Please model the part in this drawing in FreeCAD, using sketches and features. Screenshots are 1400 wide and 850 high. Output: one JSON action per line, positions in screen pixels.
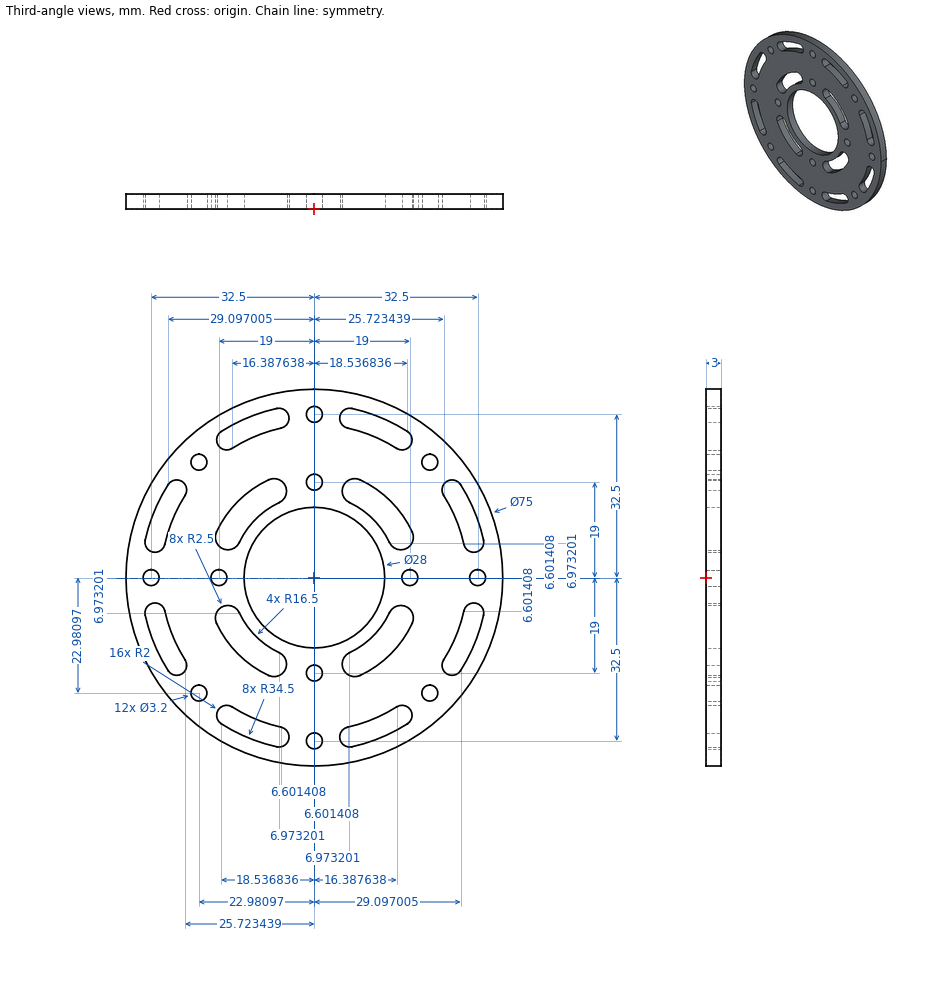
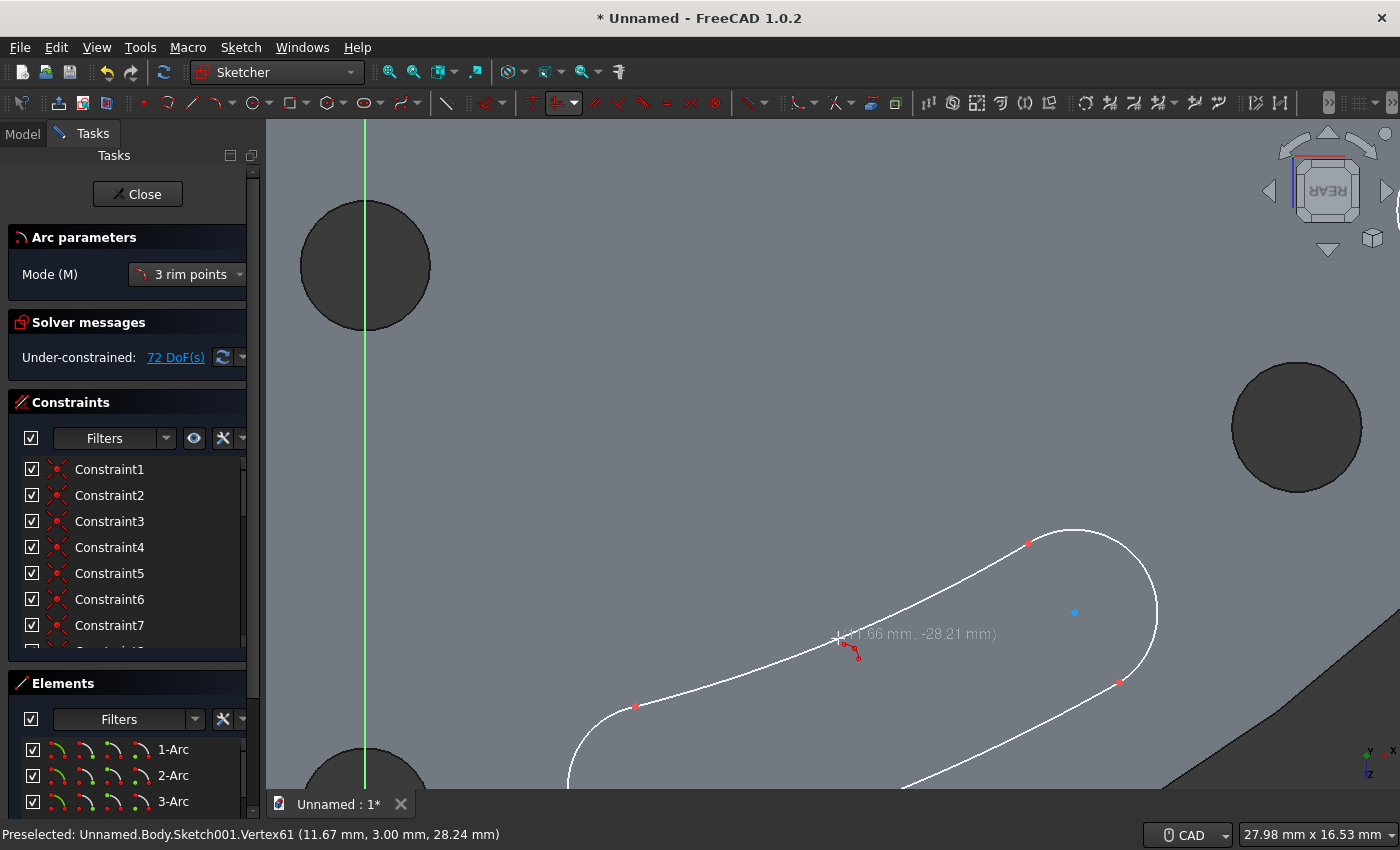
{"action": "scroll", "coordinate": [844, 644], "scroll_direction": "down", "scroll_amount": 9}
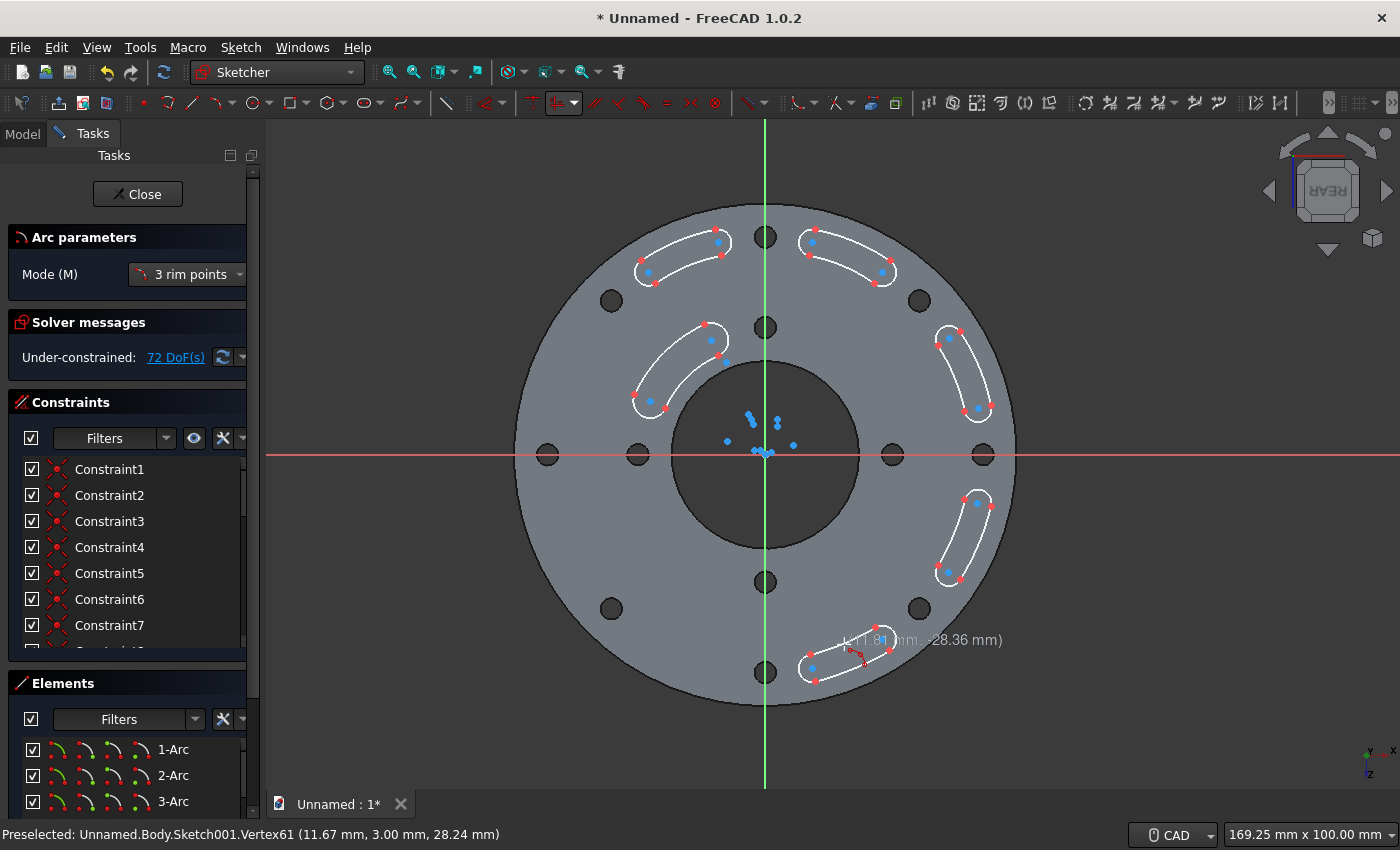
{"action": "left_click", "coordinate": [721, 654]}
{"action": "left_click", "coordinate": [656, 627]}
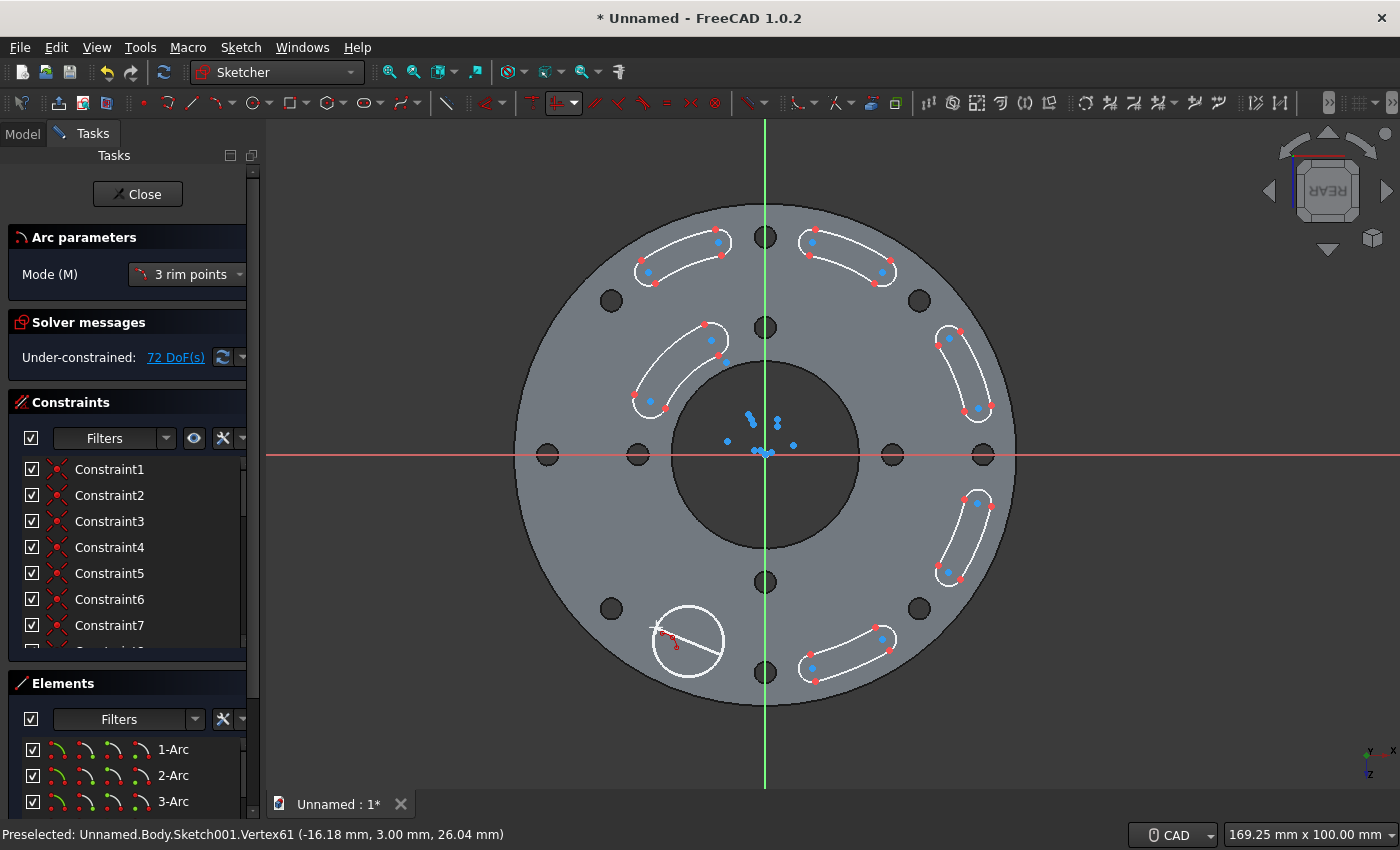
{"action": "scroll", "coordinate": [687, 644], "scroll_direction": "up", "scroll_amount": 9}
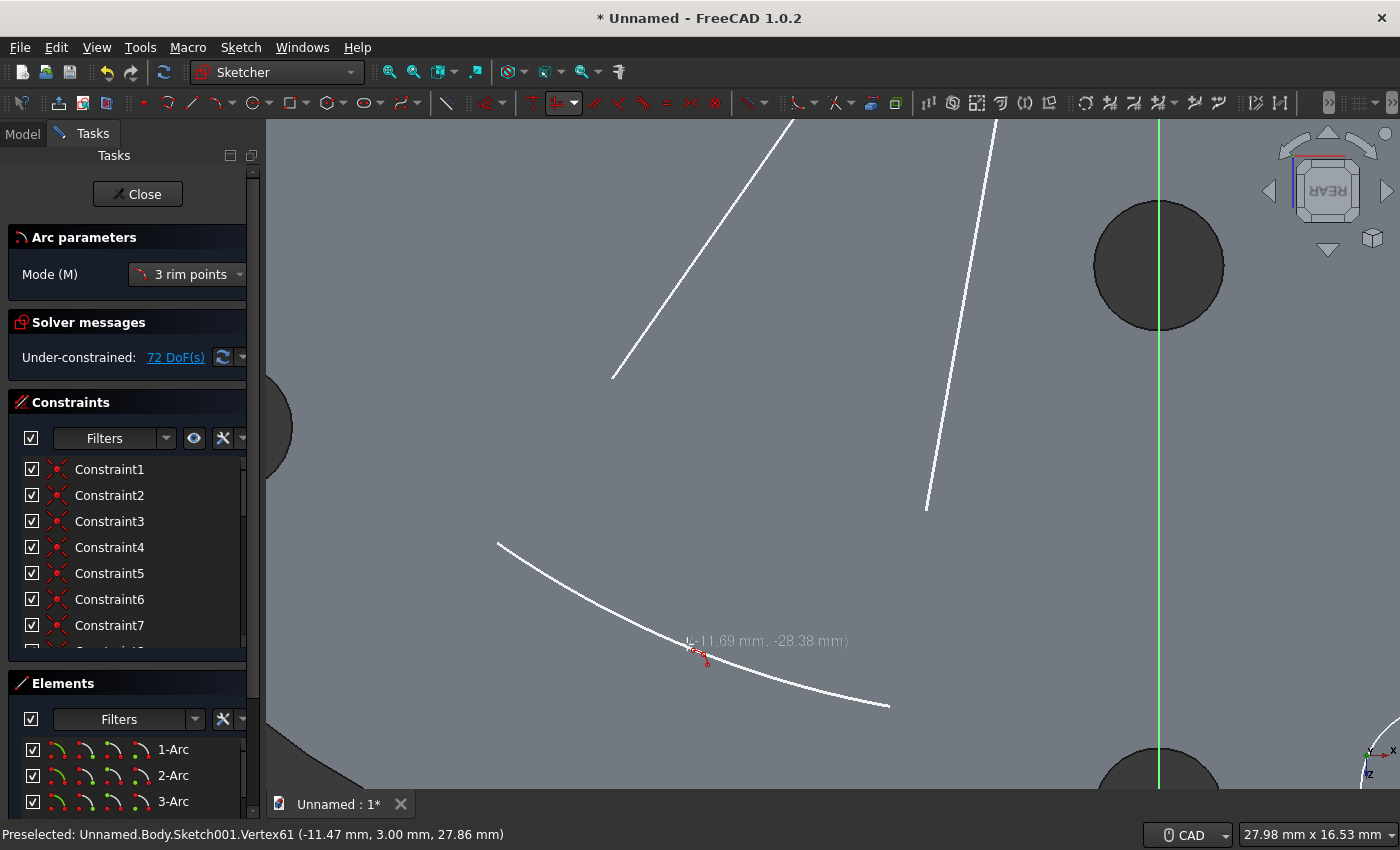
{"action": "left_click", "coordinate": [686, 638]}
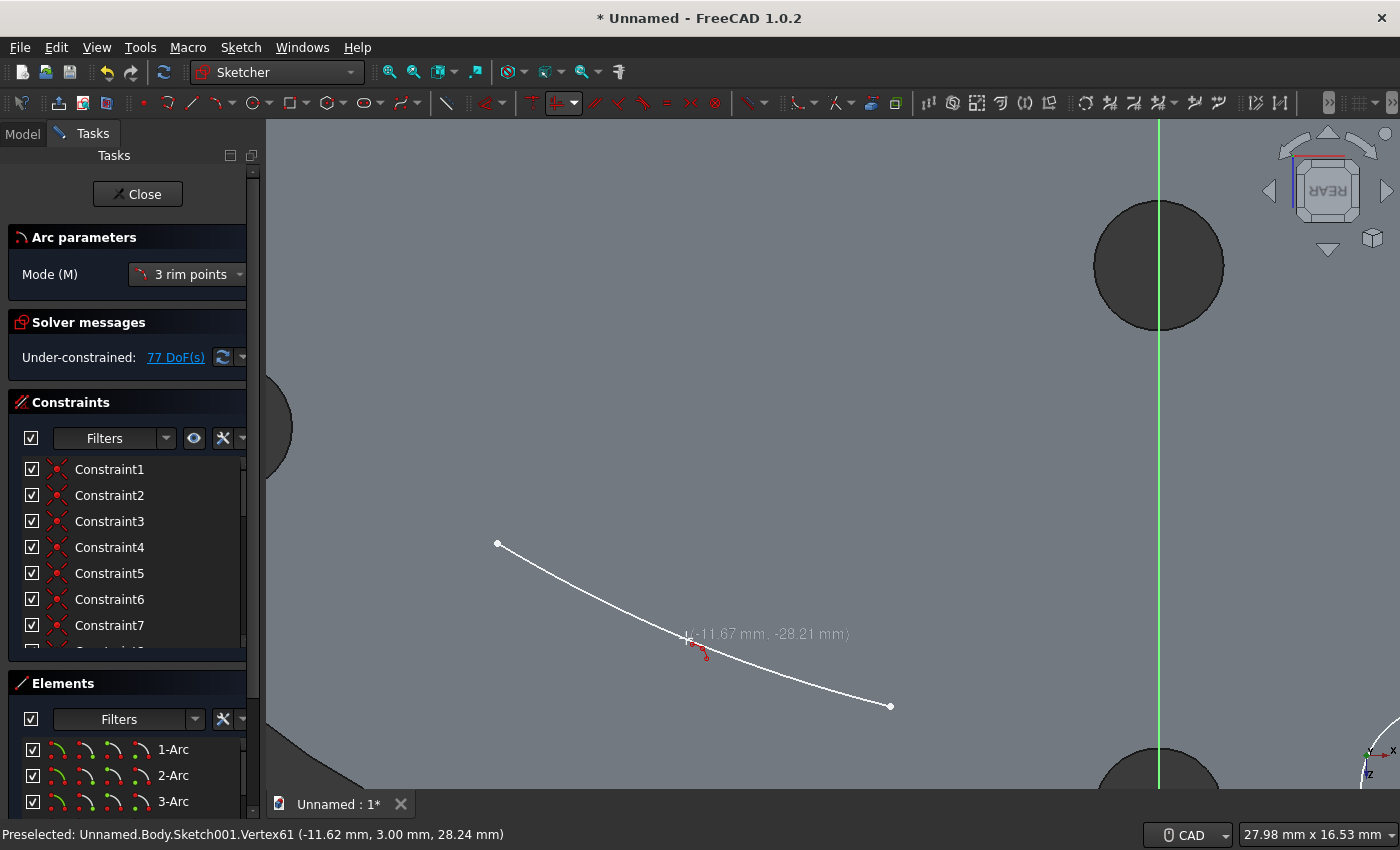
{"action": "scroll", "coordinate": [686, 644], "scroll_direction": "down", "scroll_amount": 9}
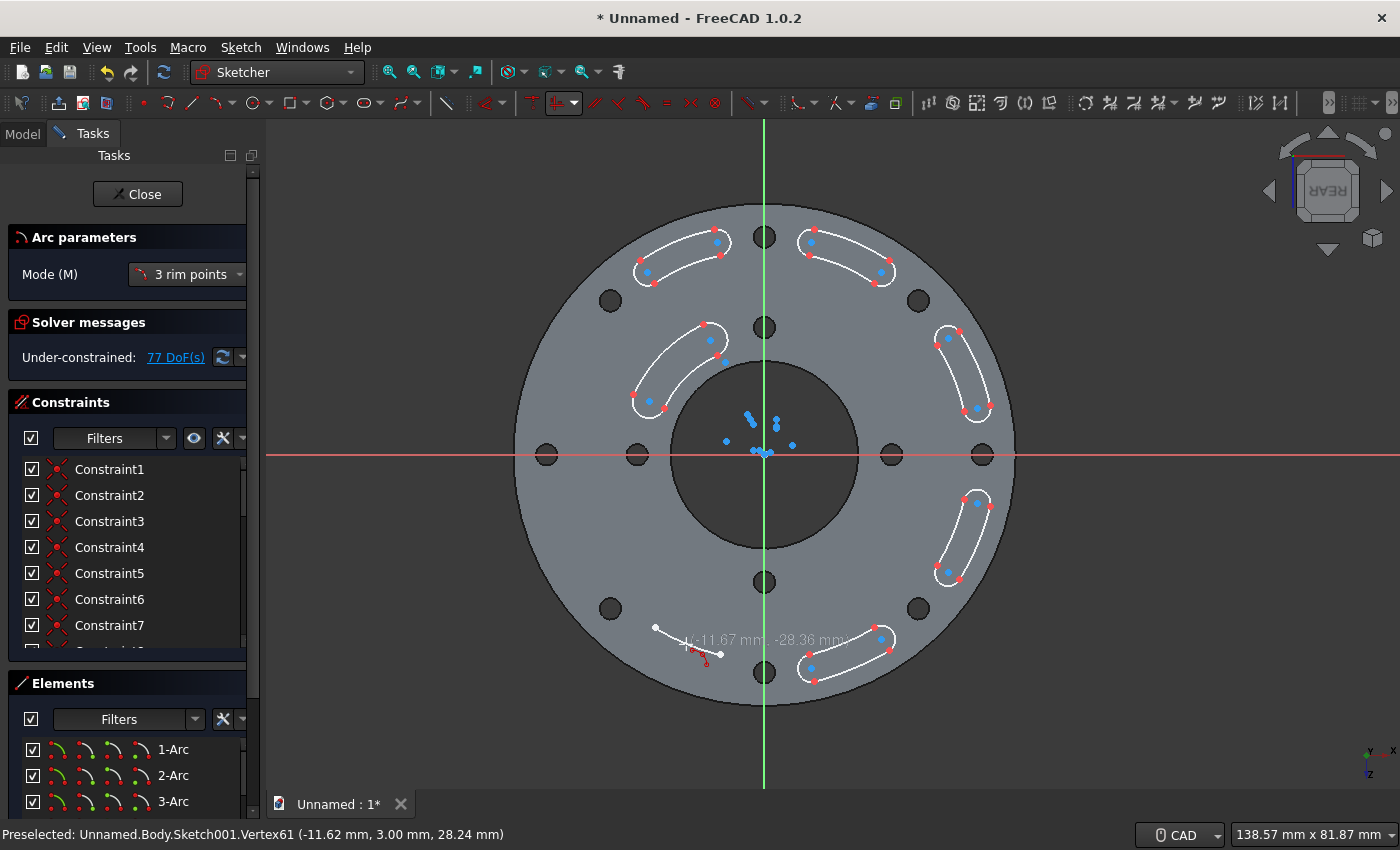
{"action": "left_click", "coordinate": [655, 628]}
{"action": "left_click", "coordinate": [640, 650]}
{"action": "left_click", "coordinate": [636, 631]}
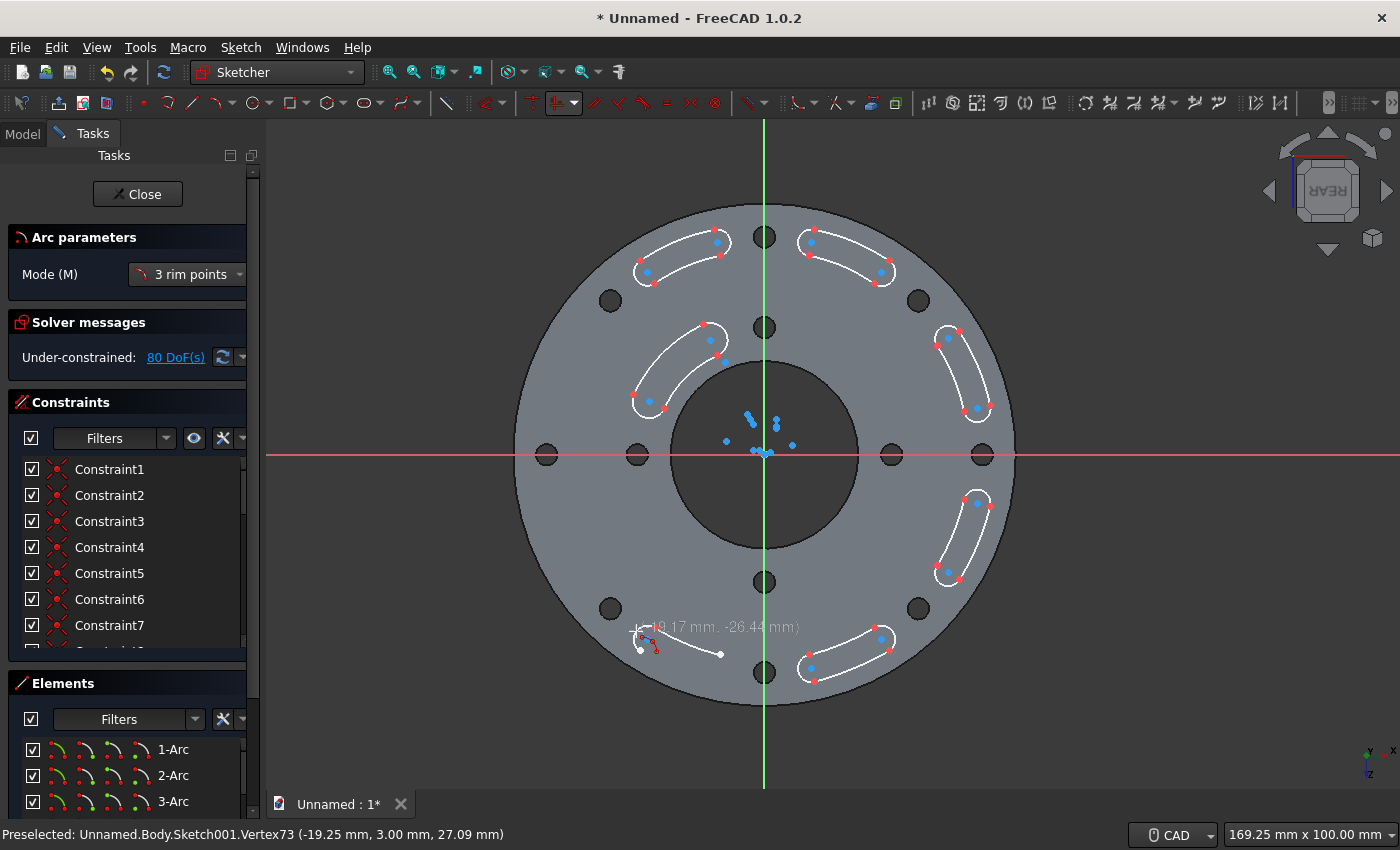
{"action": "left_click", "coordinate": [640, 651]}
{"action": "left_click", "coordinate": [714, 681]}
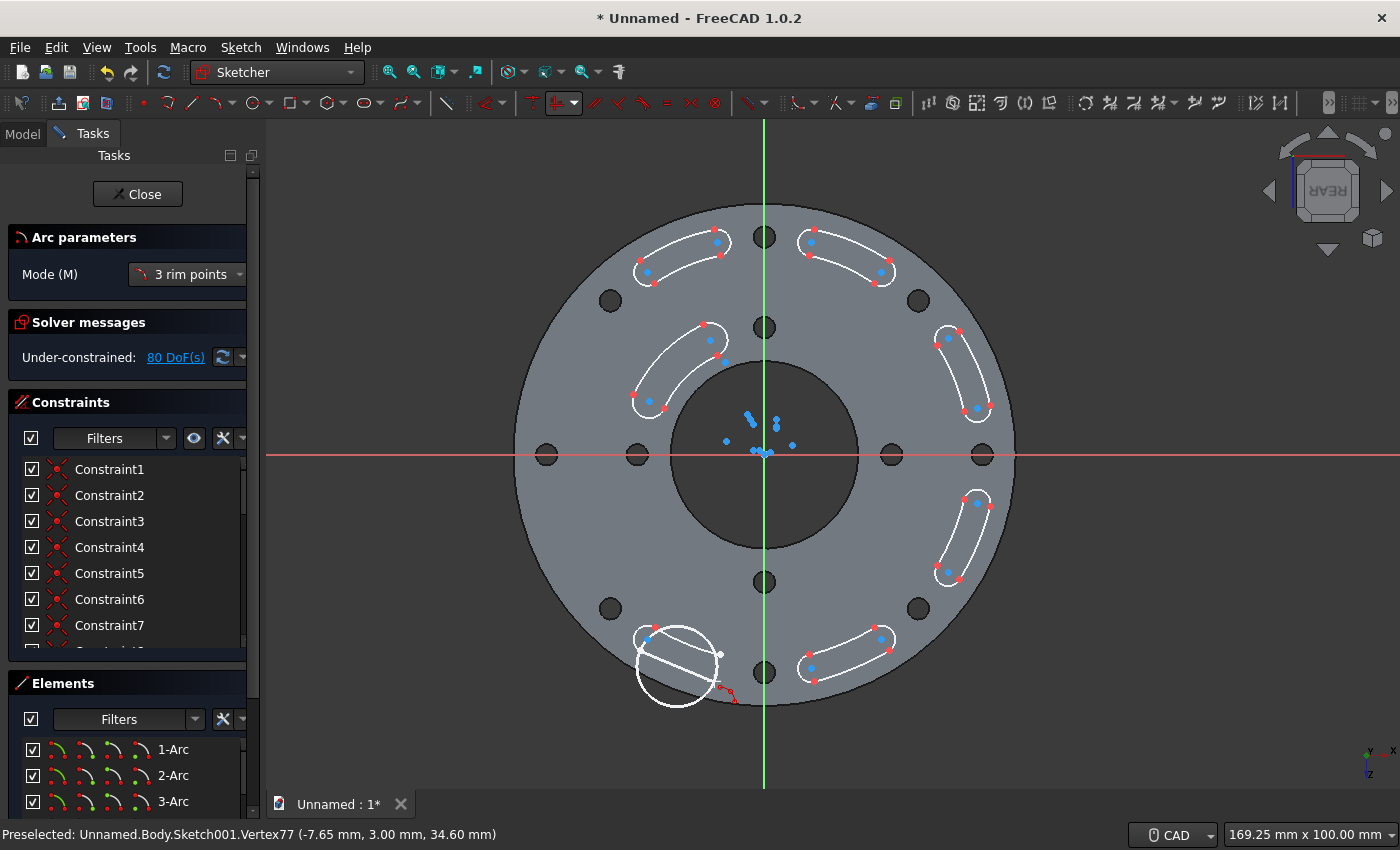
{"action": "scroll", "coordinate": [676, 668], "scroll_direction": "up", "scroll_amount": 8}